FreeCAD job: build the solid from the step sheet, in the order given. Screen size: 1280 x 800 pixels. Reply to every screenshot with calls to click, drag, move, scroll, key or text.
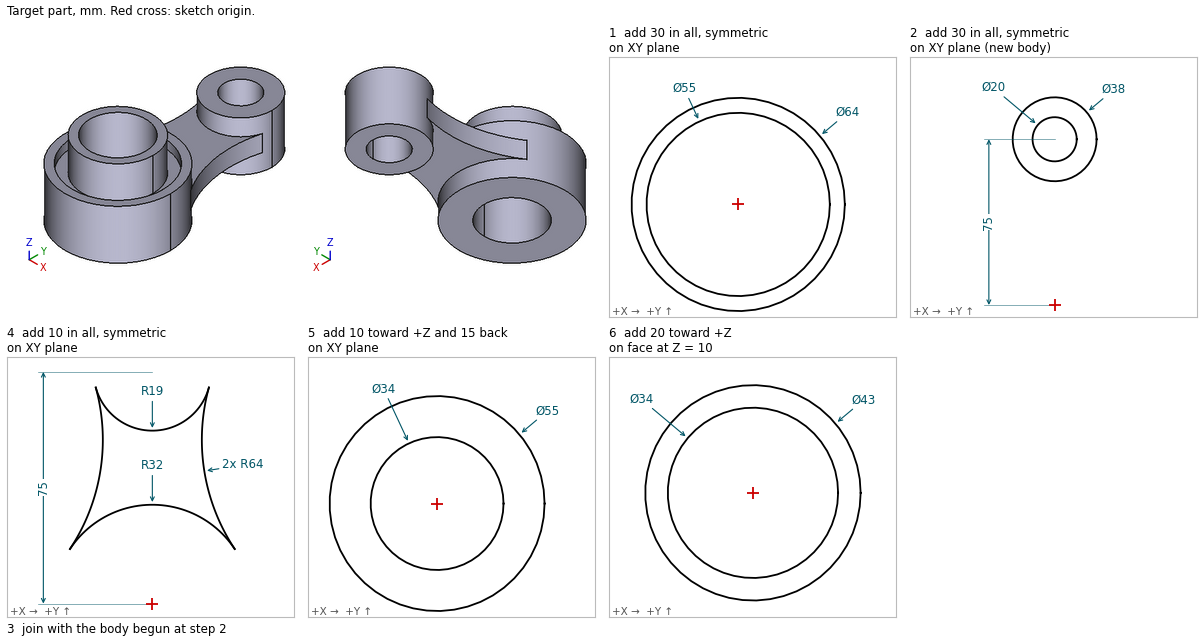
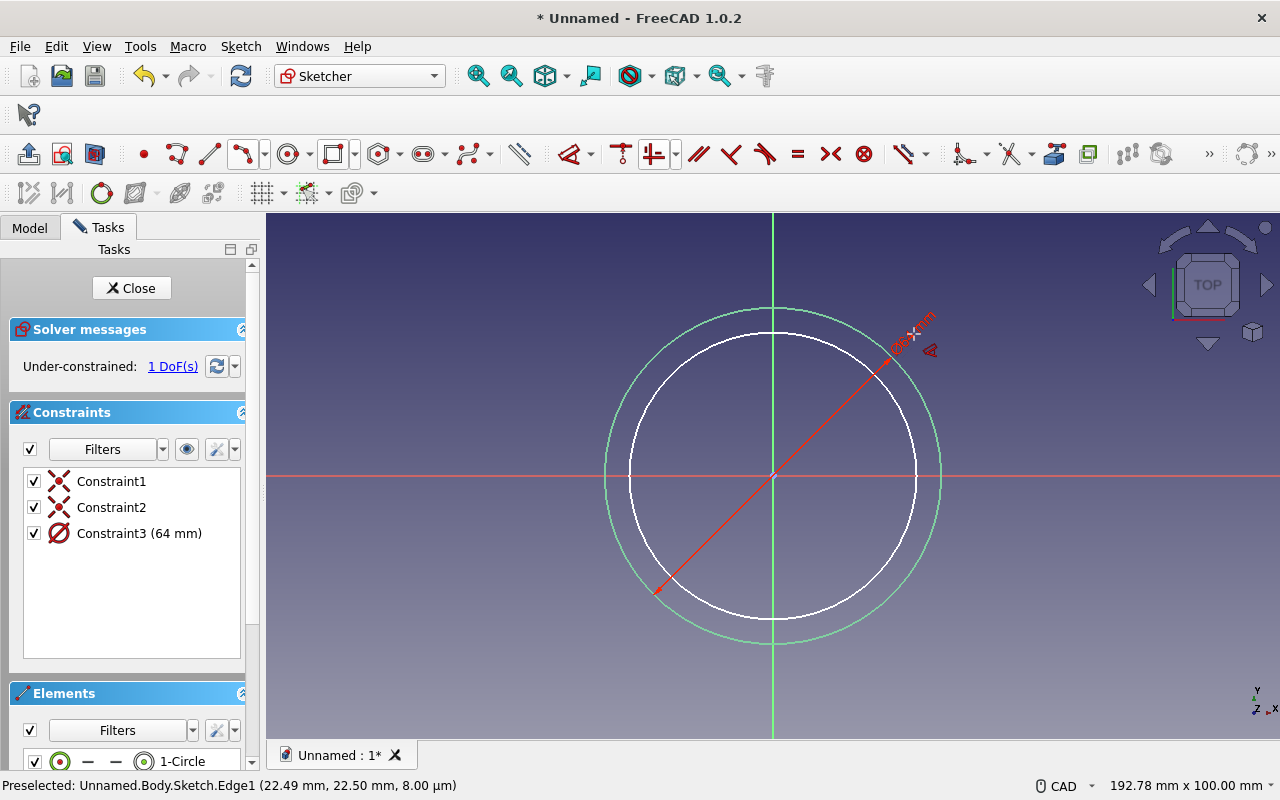
click(874, 374)
click(963, 419)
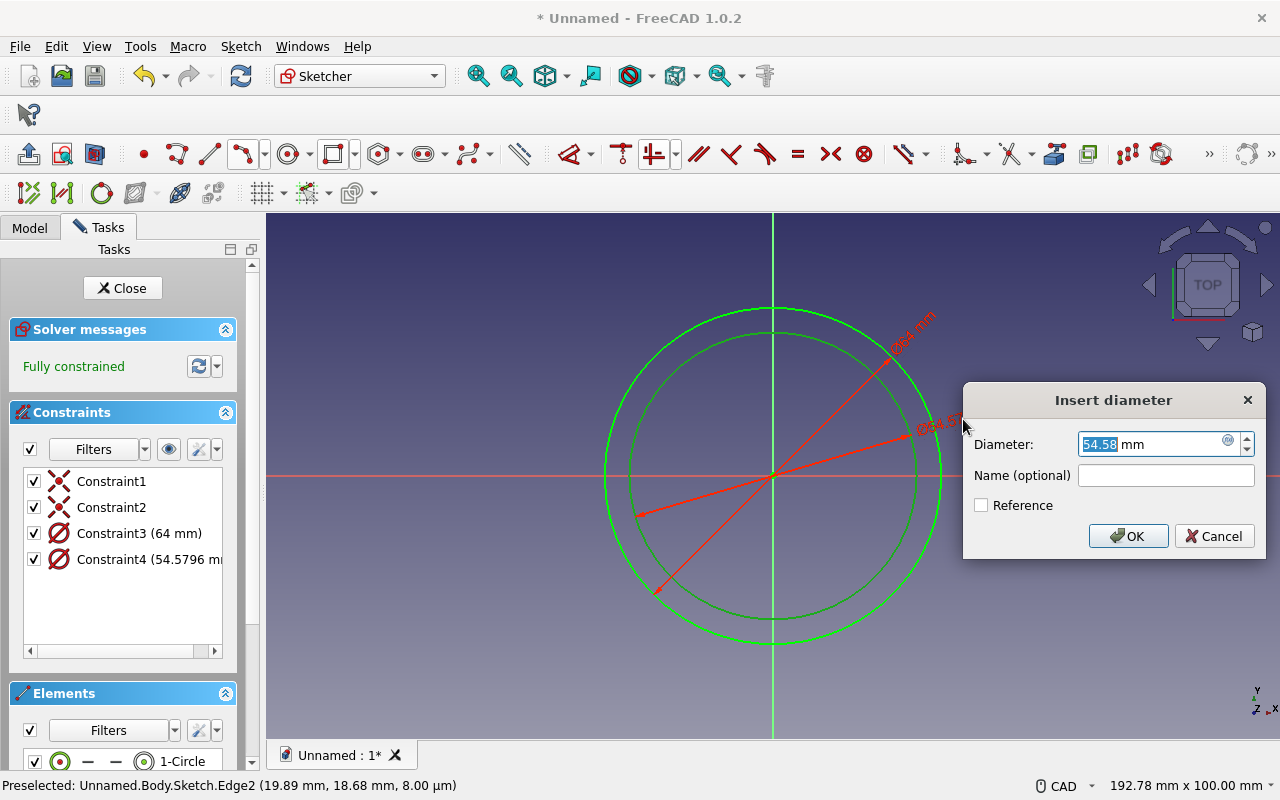
text(55)
key(Return)
key(Escape)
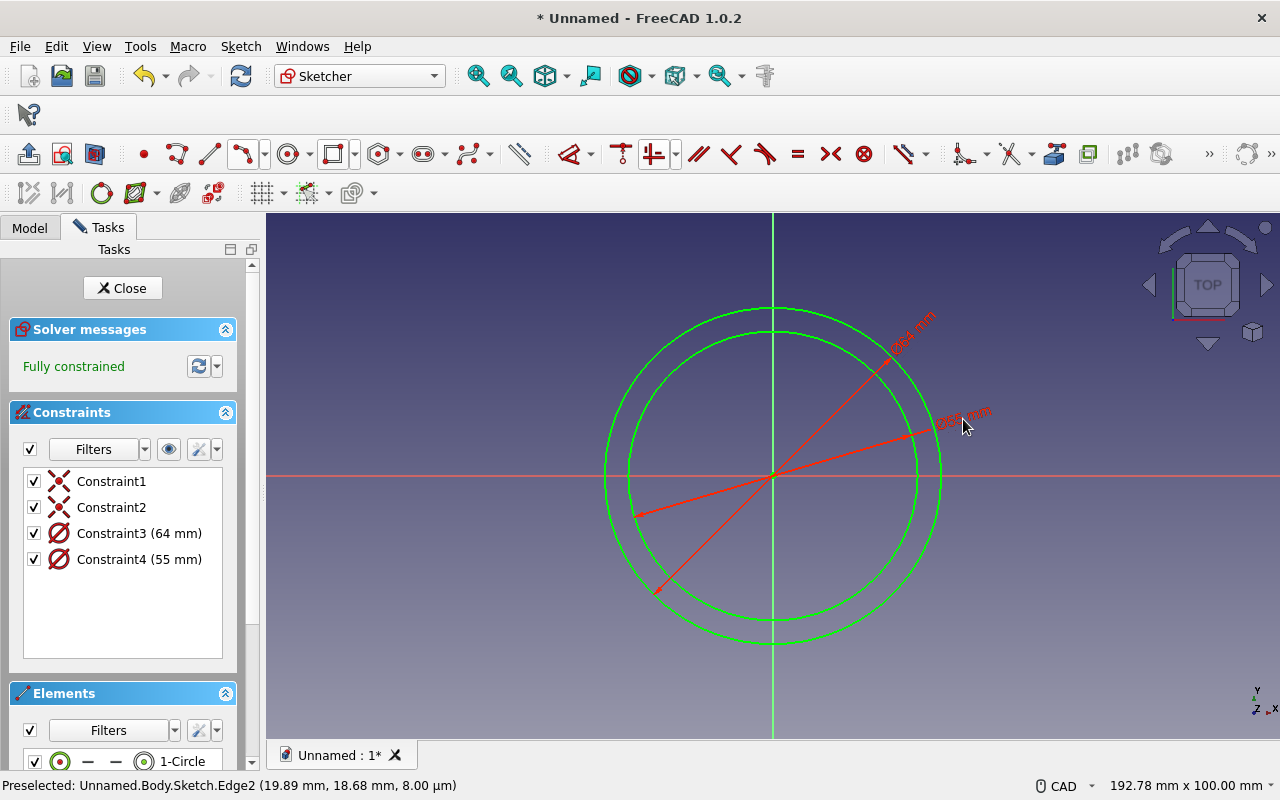
click(123, 288)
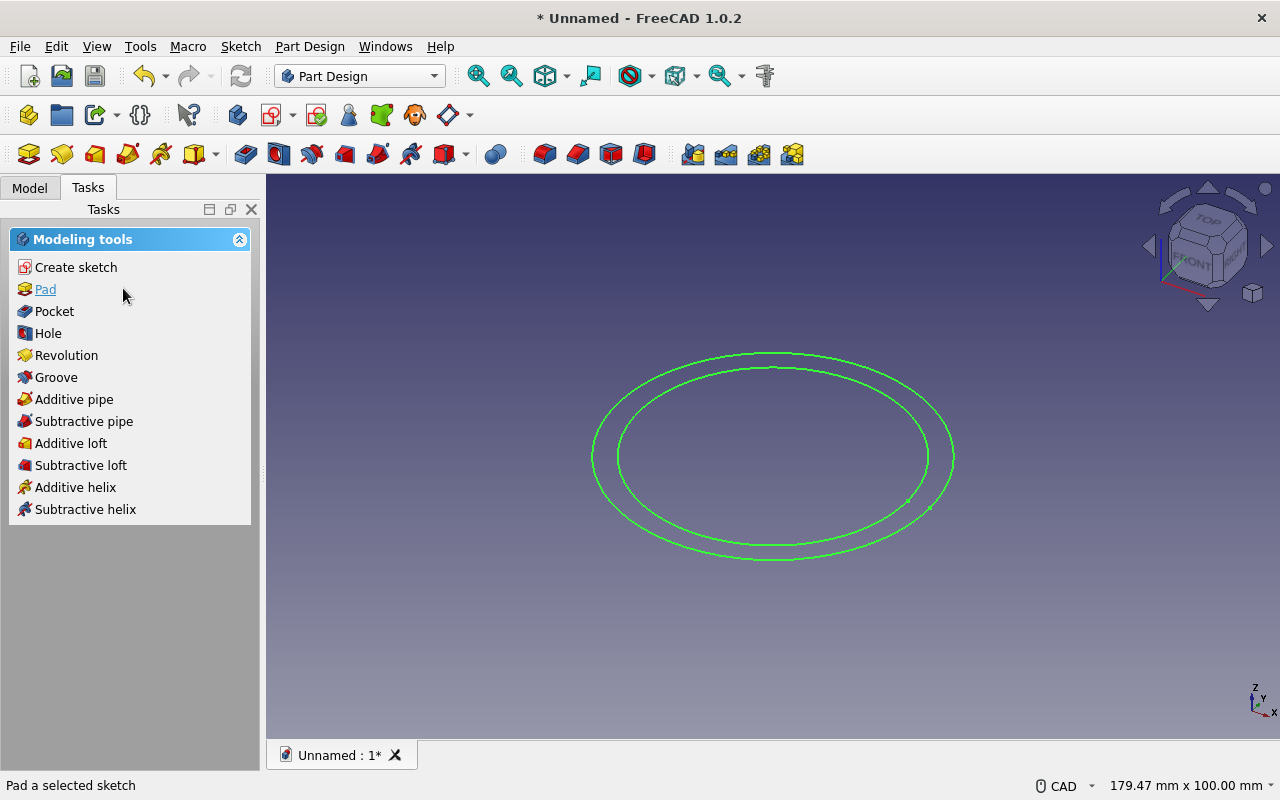
click(29, 154)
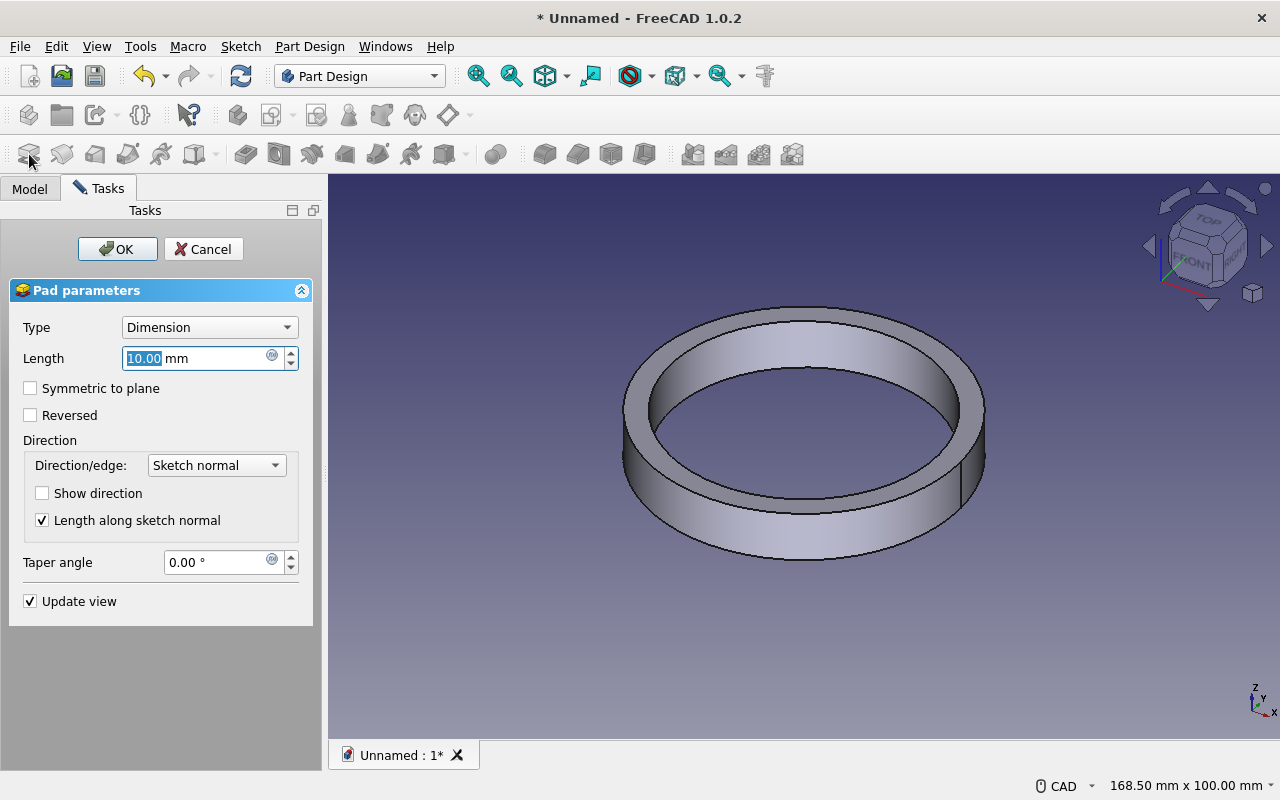
text(30)
key(Tab)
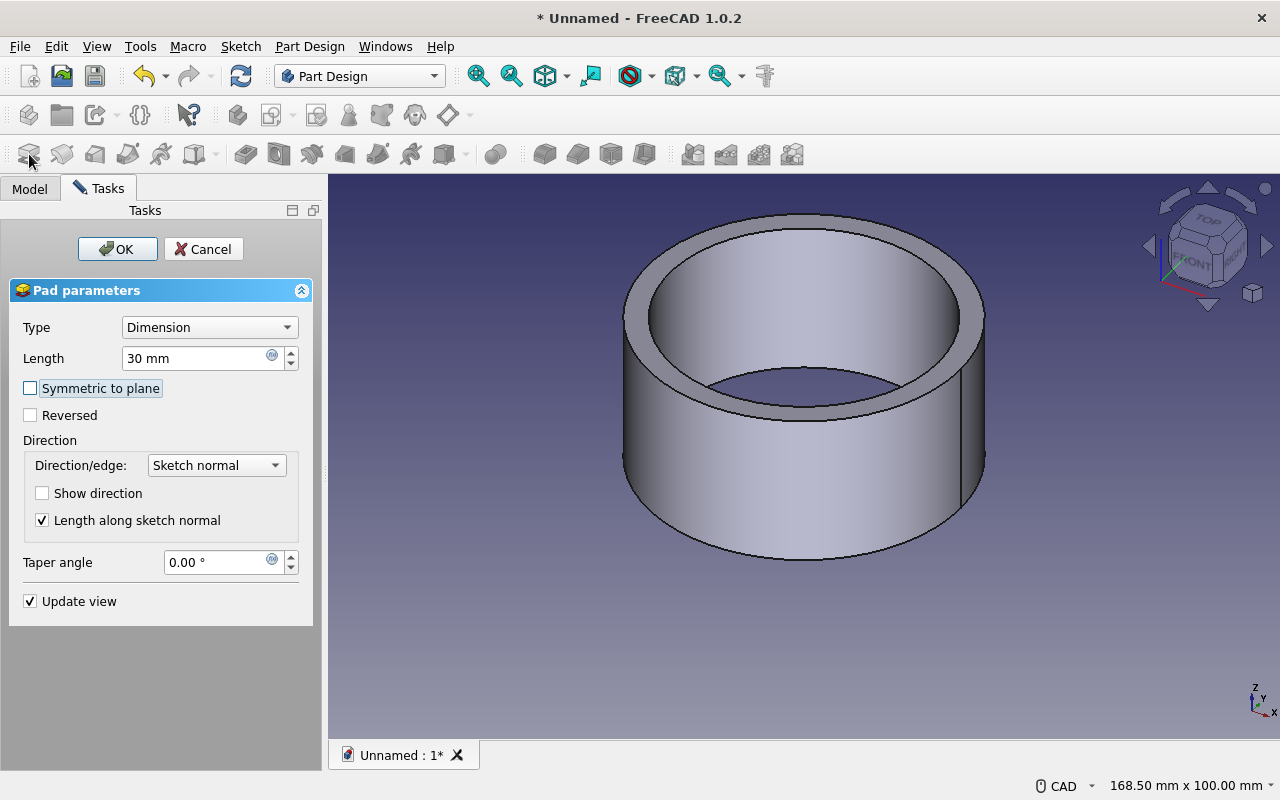
click(31, 388)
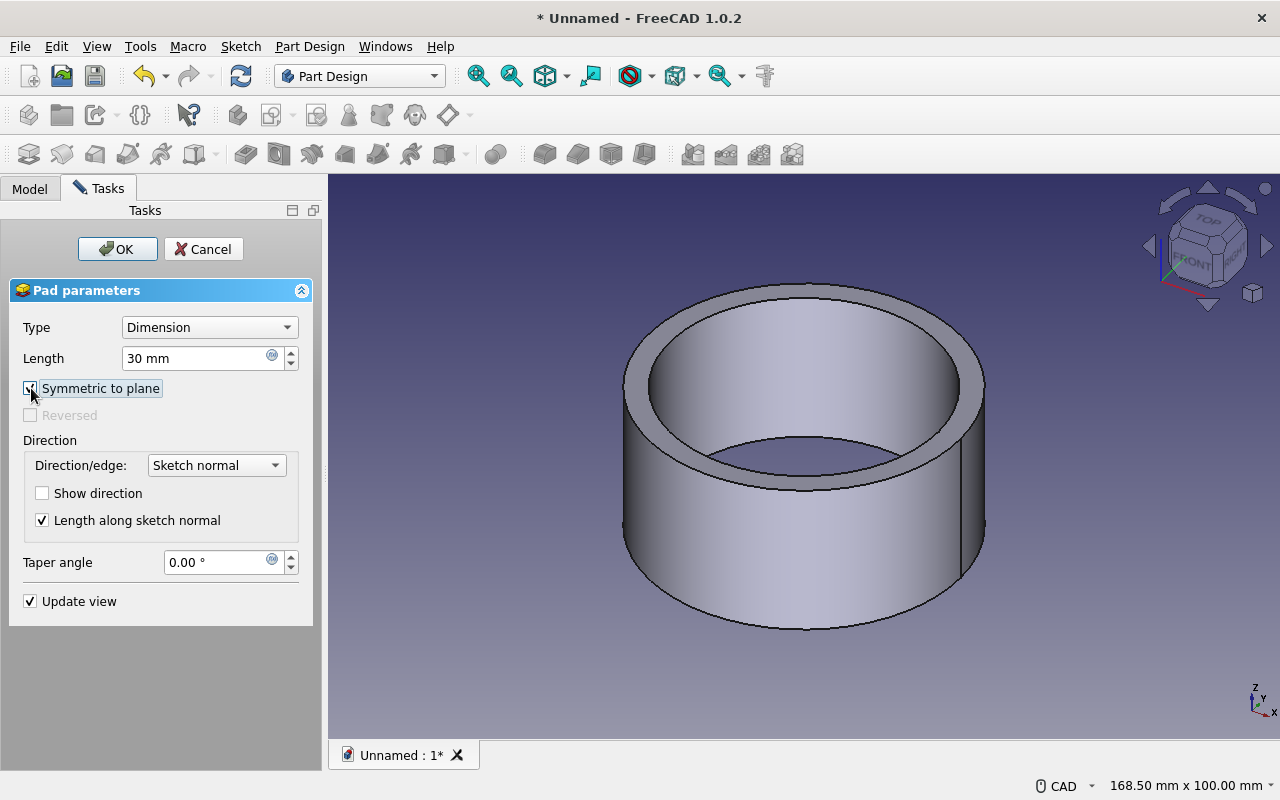
click(118, 249)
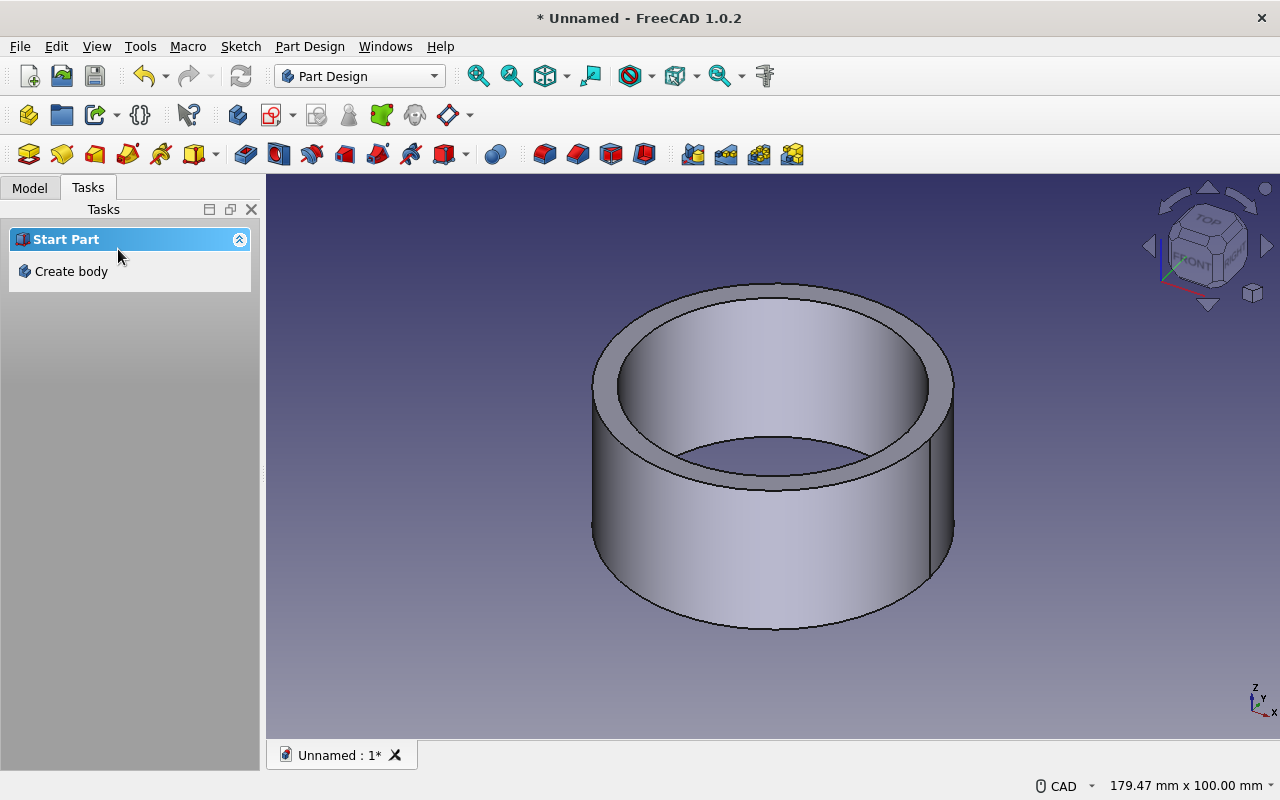
click(238, 116)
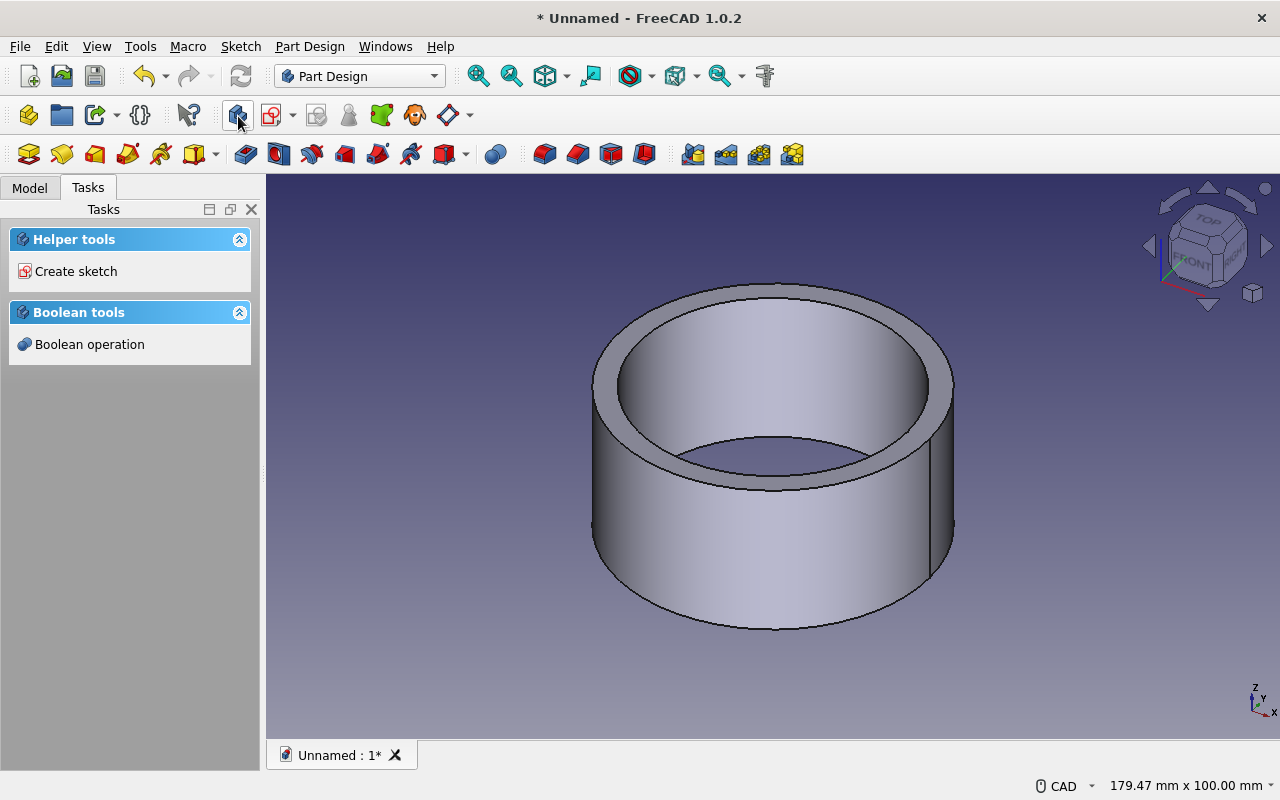
click(306, 699)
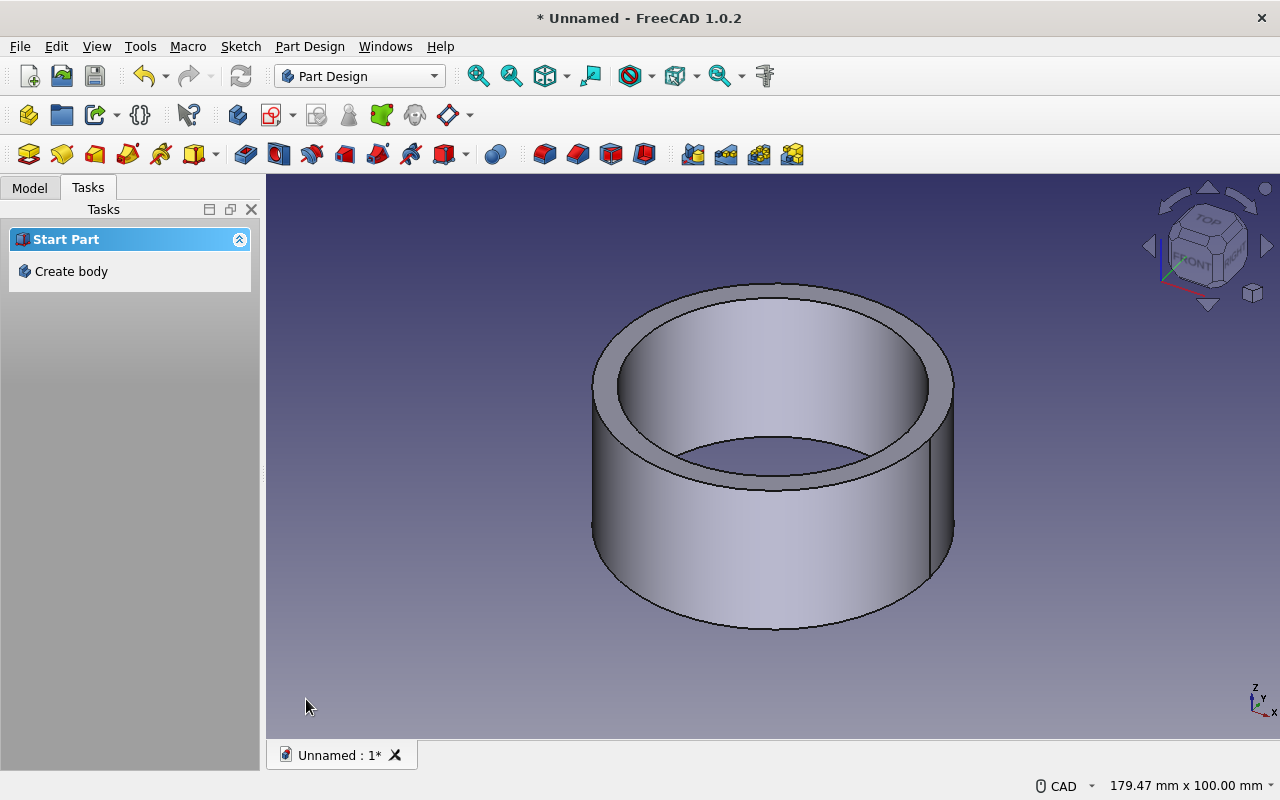
click(270, 116)